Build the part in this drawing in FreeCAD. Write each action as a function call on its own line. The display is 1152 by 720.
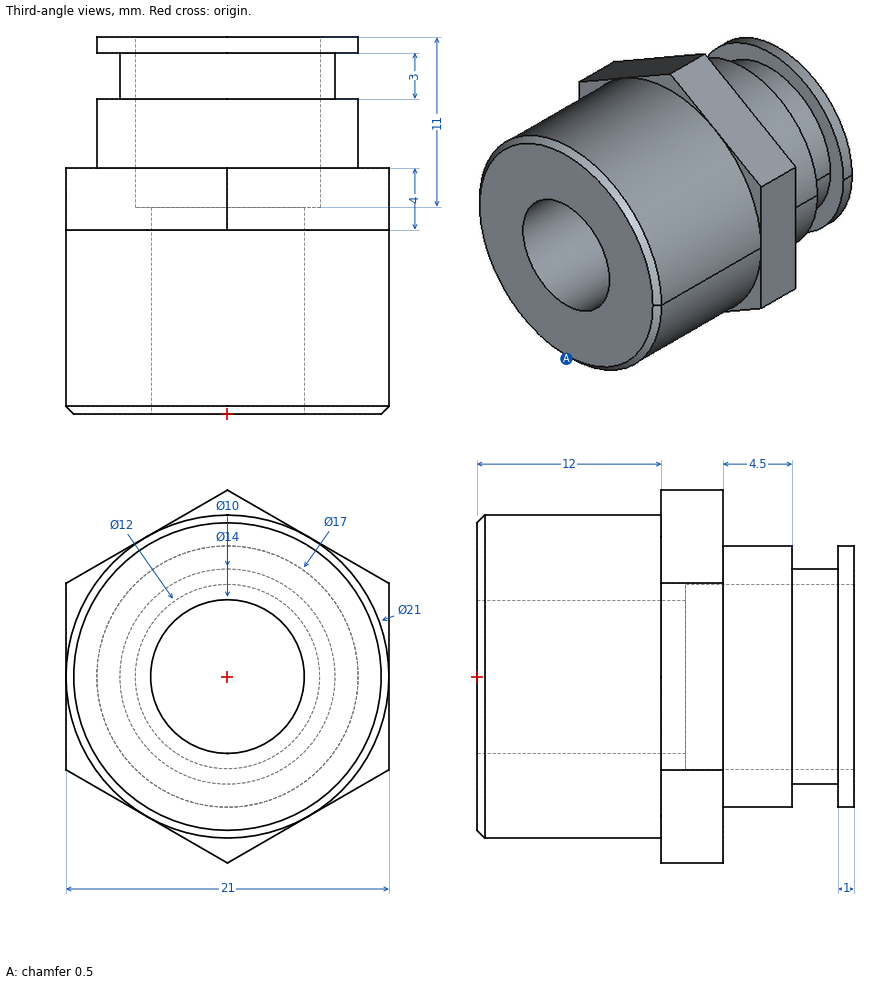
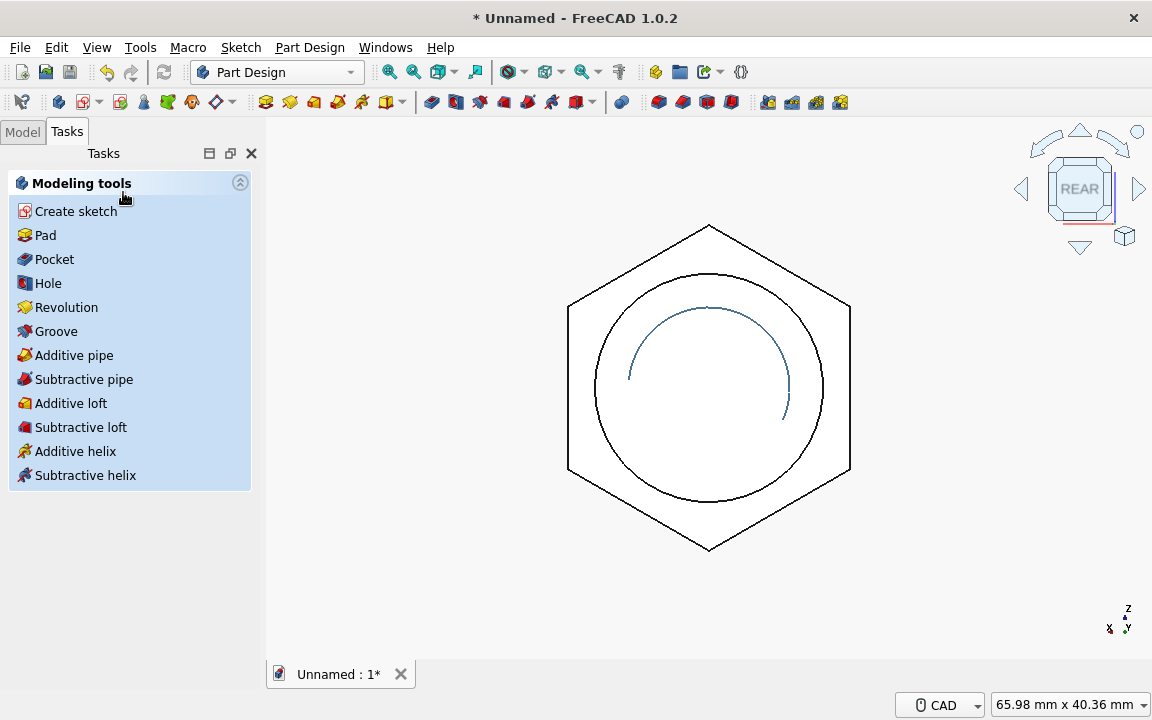
click(432, 102)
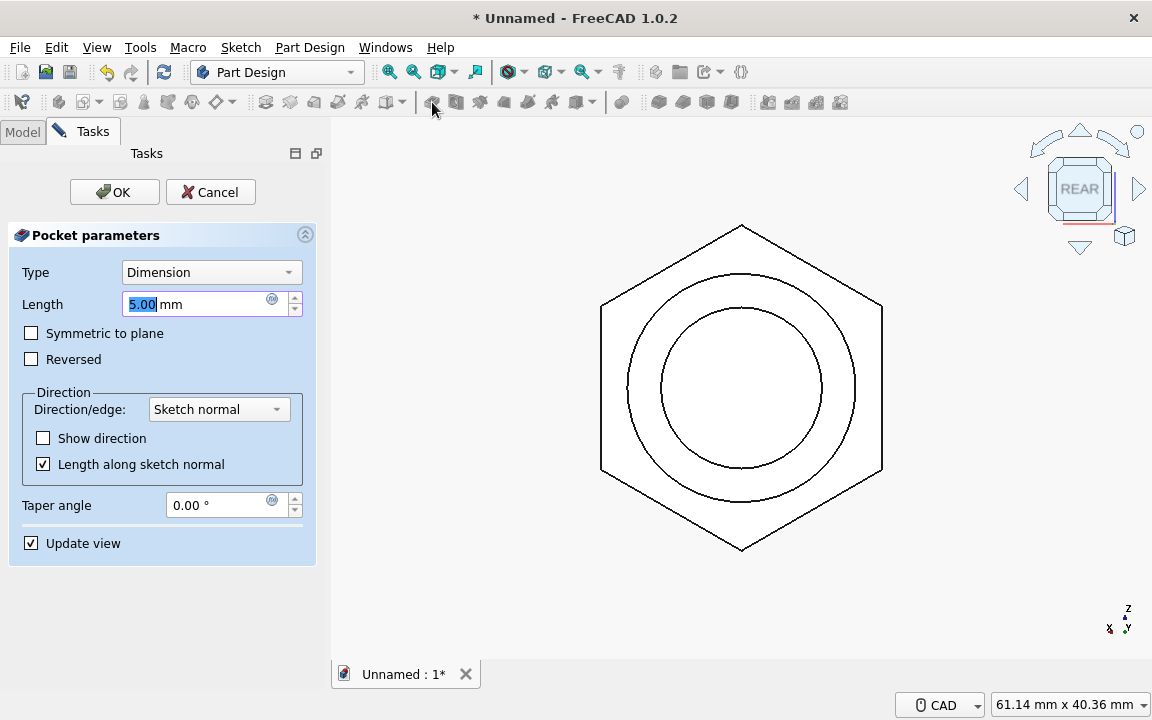
text(11)
key(Tab)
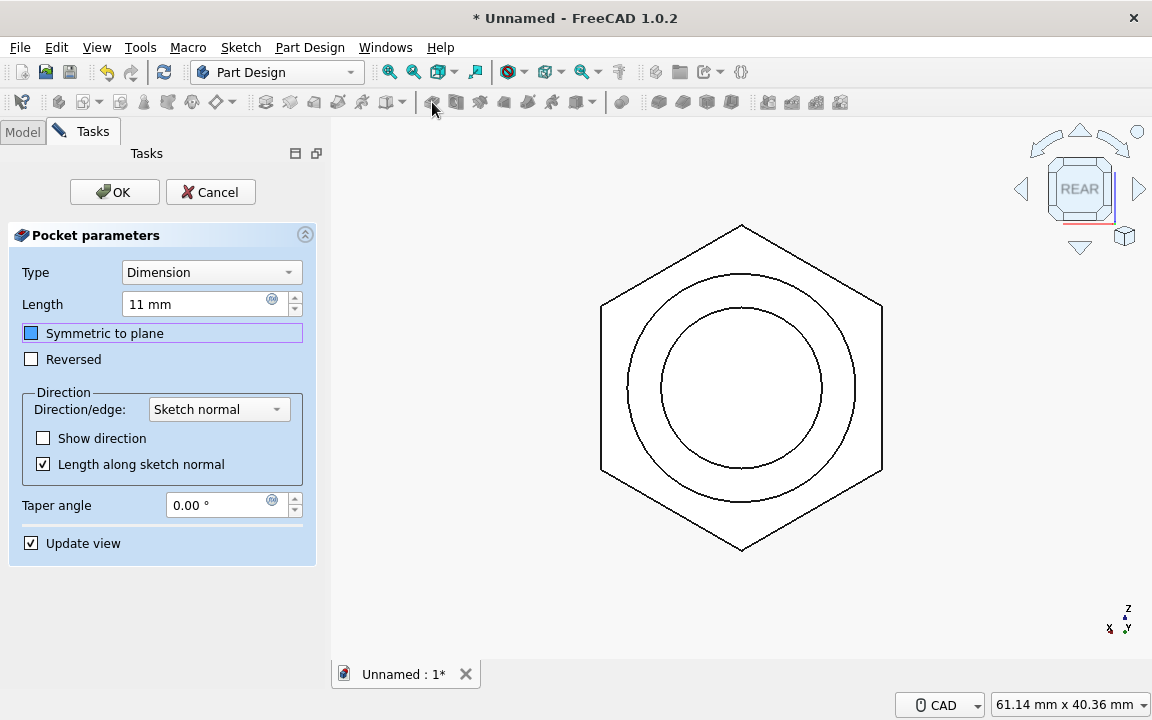
click(115, 192)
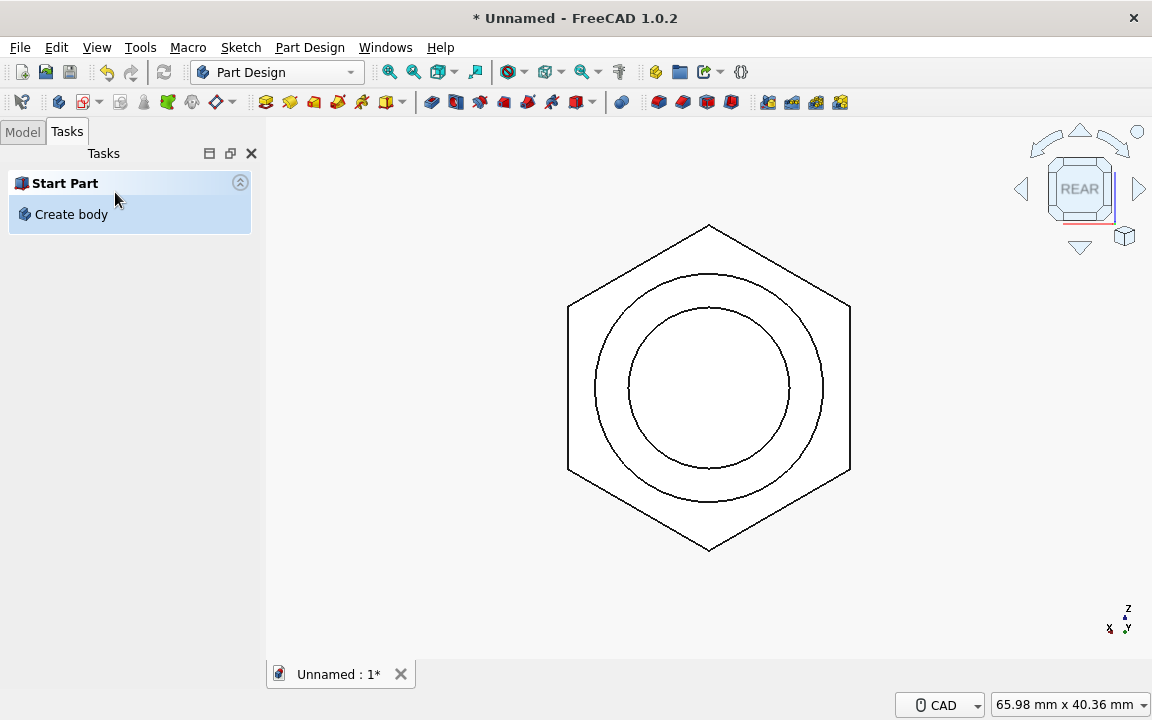
key(0)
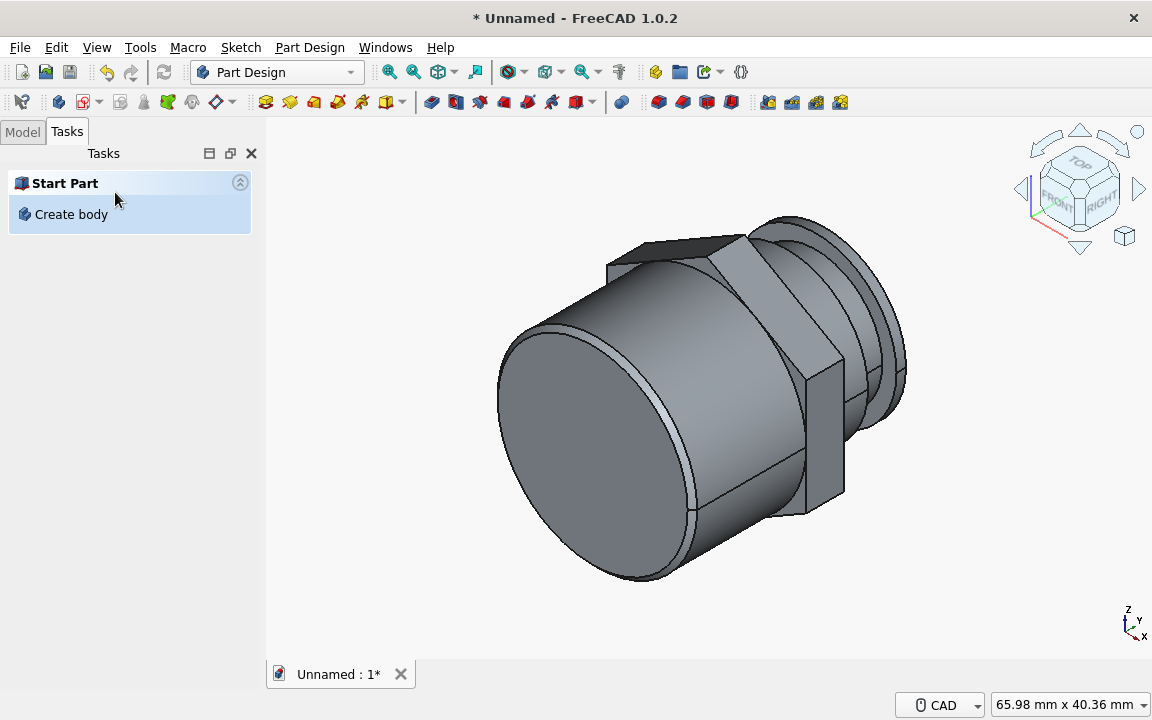
click(593, 454)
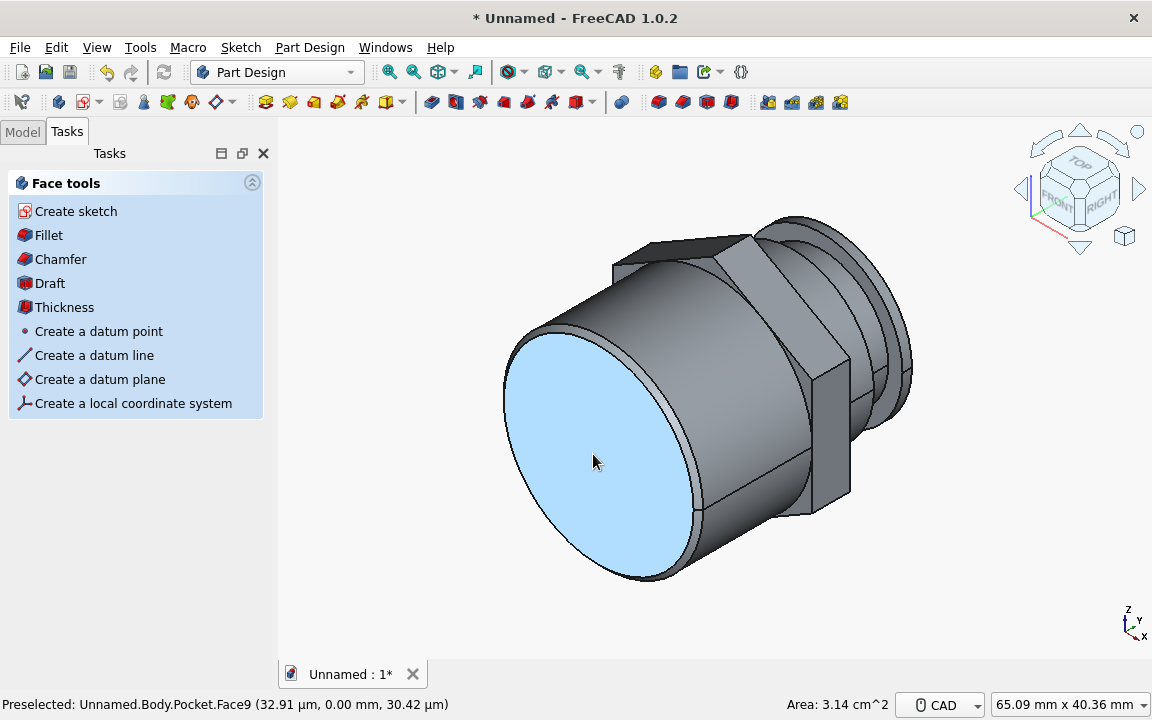
click(84, 102)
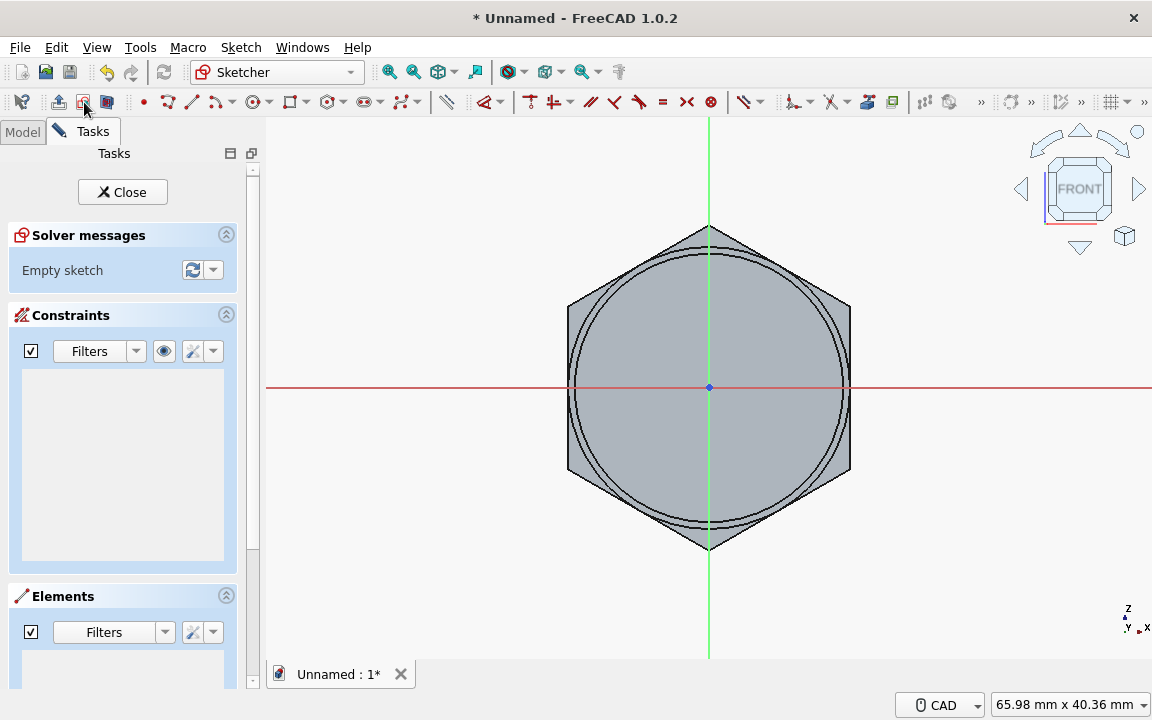
scroll(749, 388, up, 5)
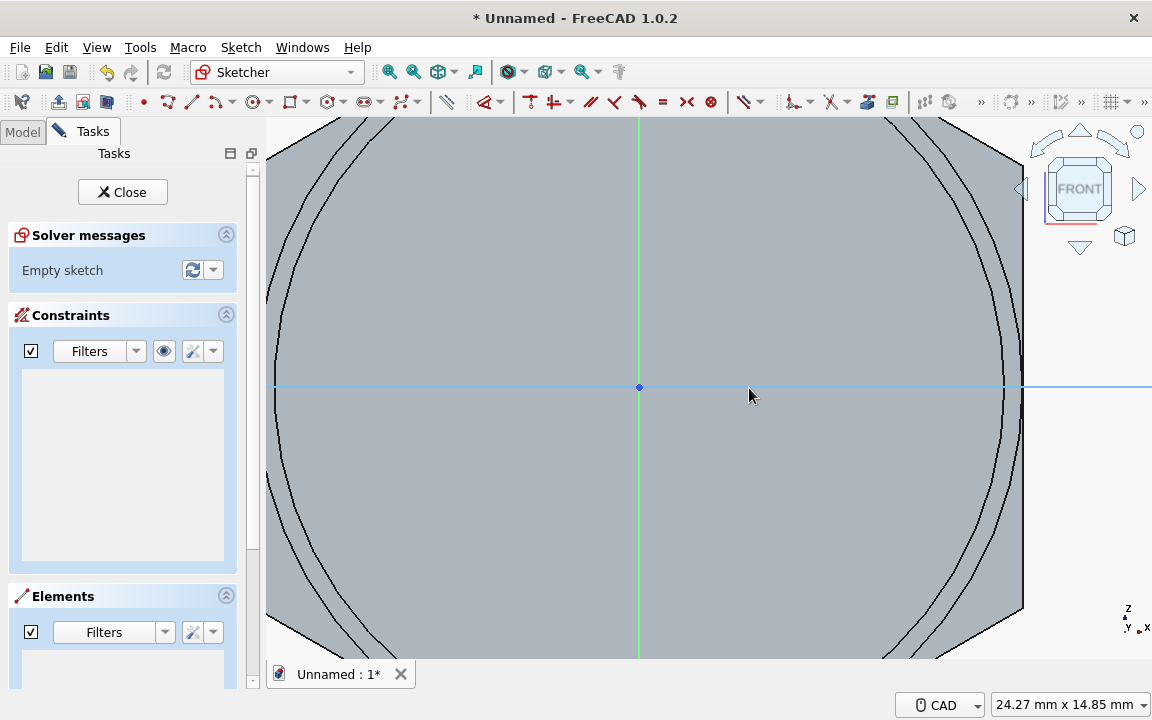
key(g)
key(c)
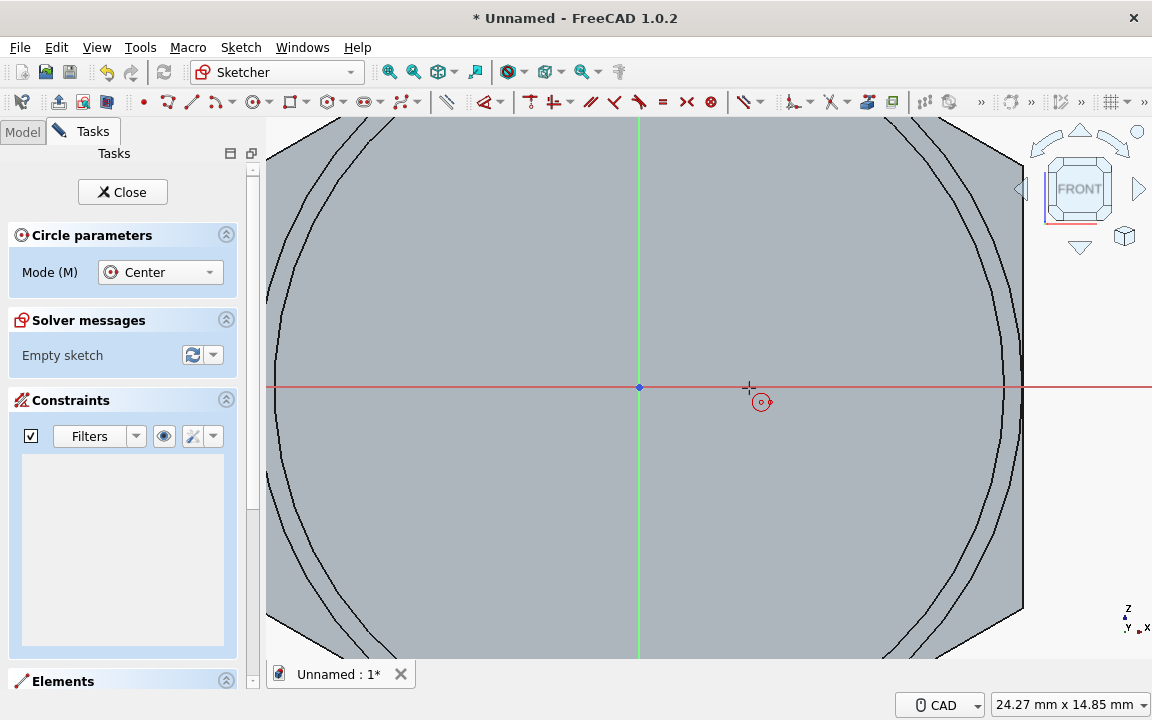
click(639, 387)
move(768, 258)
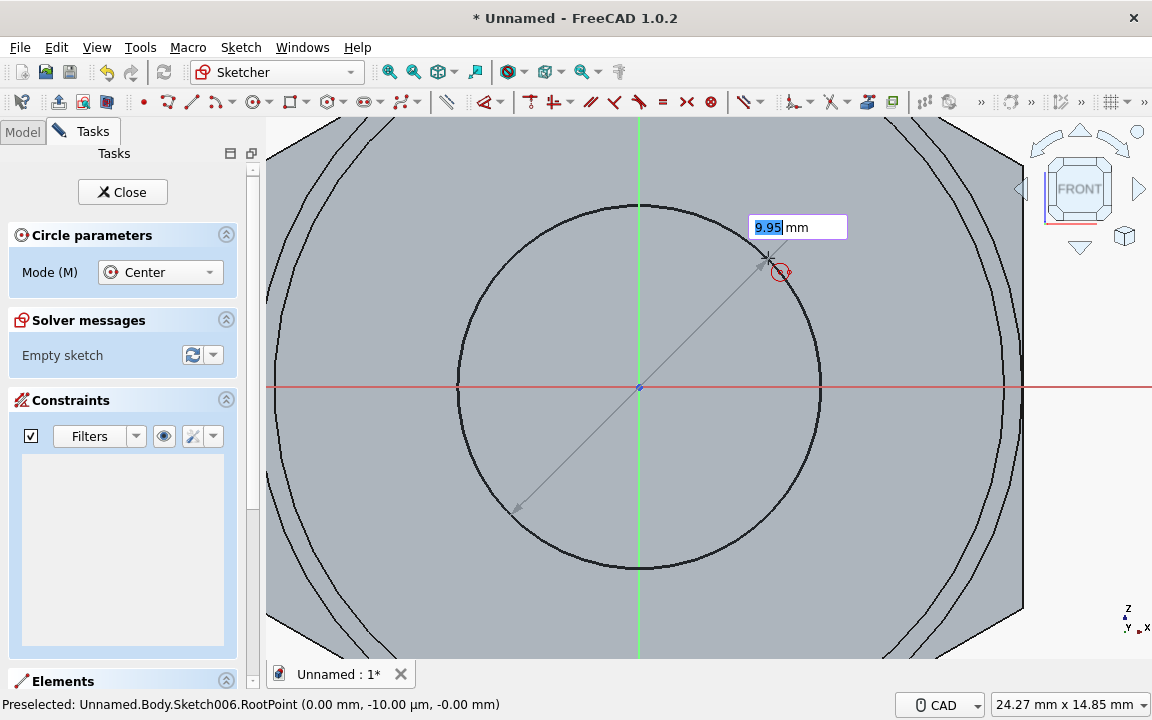
text(10)
key(Return)
key(Escape)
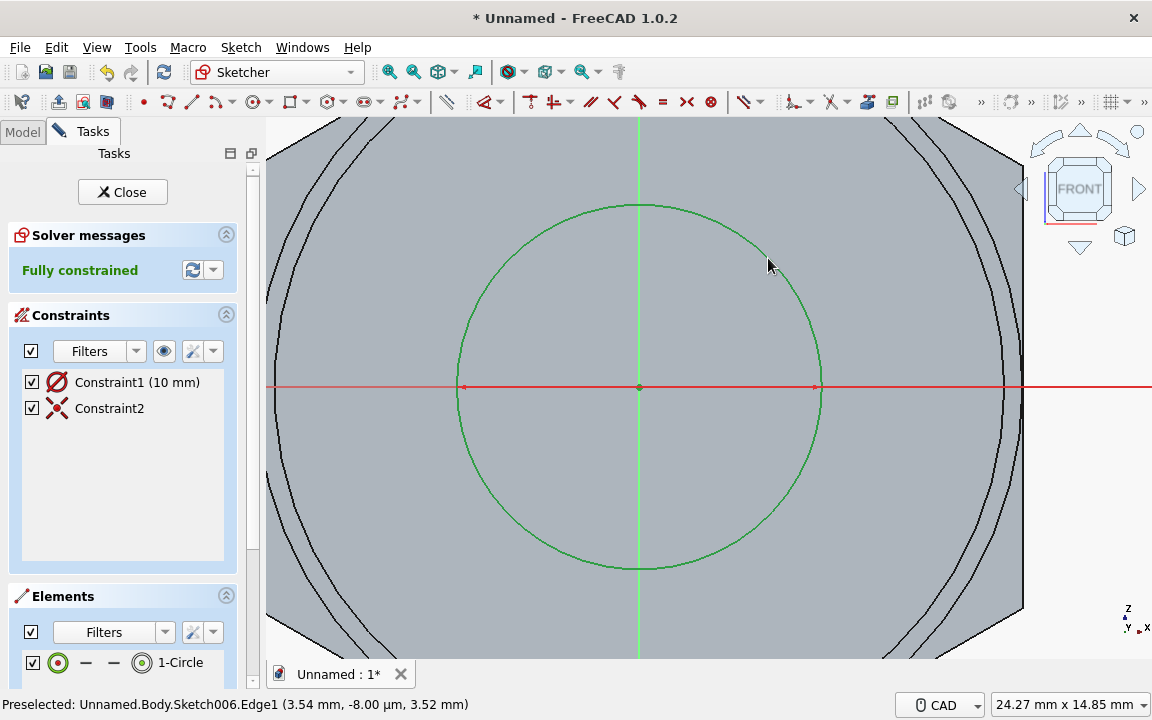
click(123, 192)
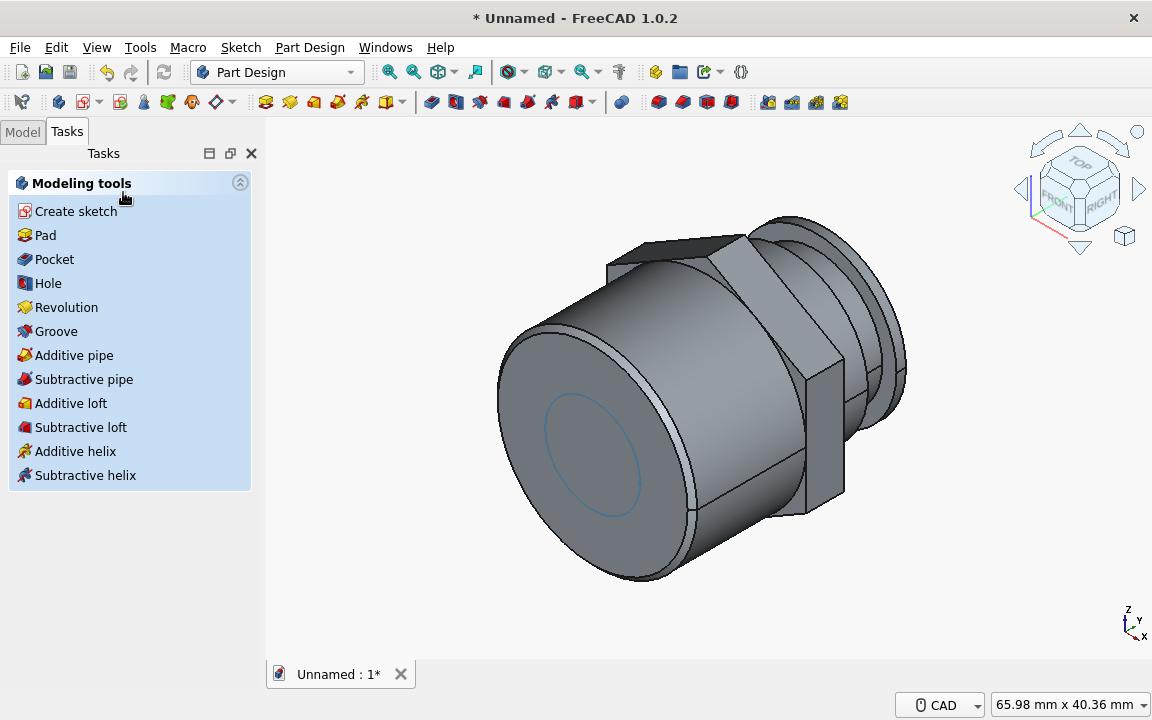
click(432, 102)